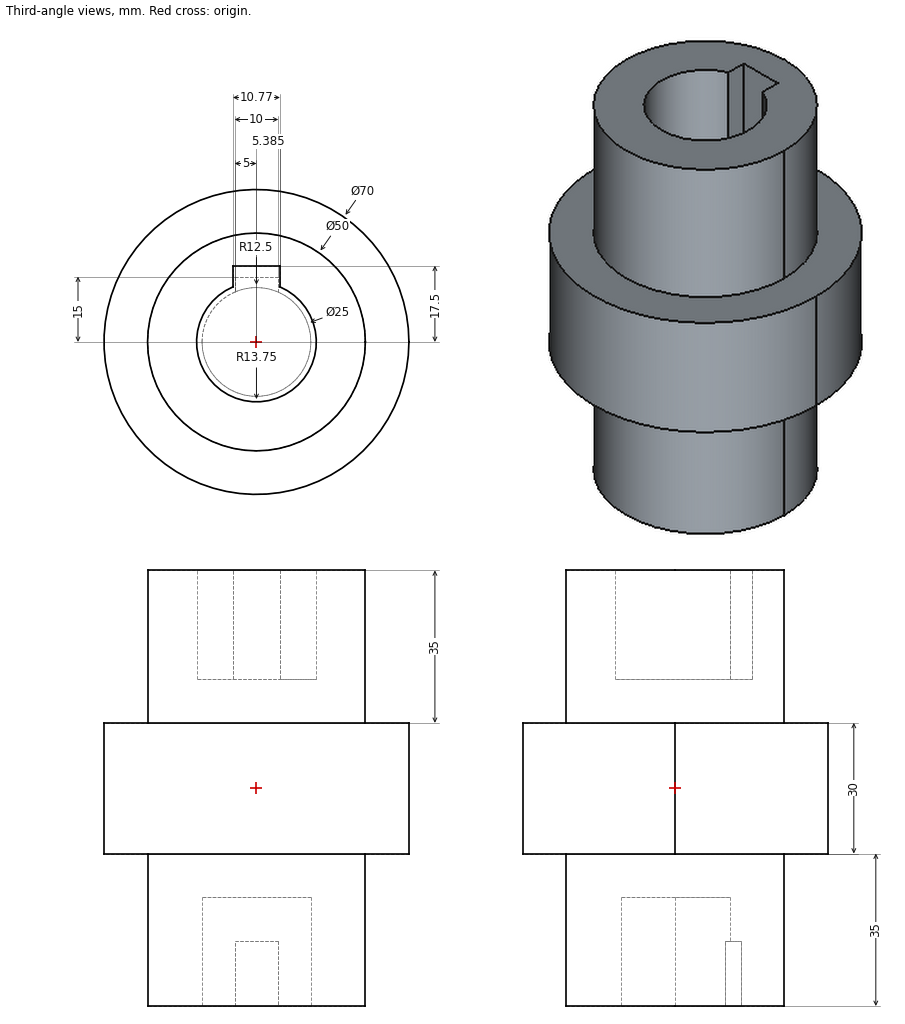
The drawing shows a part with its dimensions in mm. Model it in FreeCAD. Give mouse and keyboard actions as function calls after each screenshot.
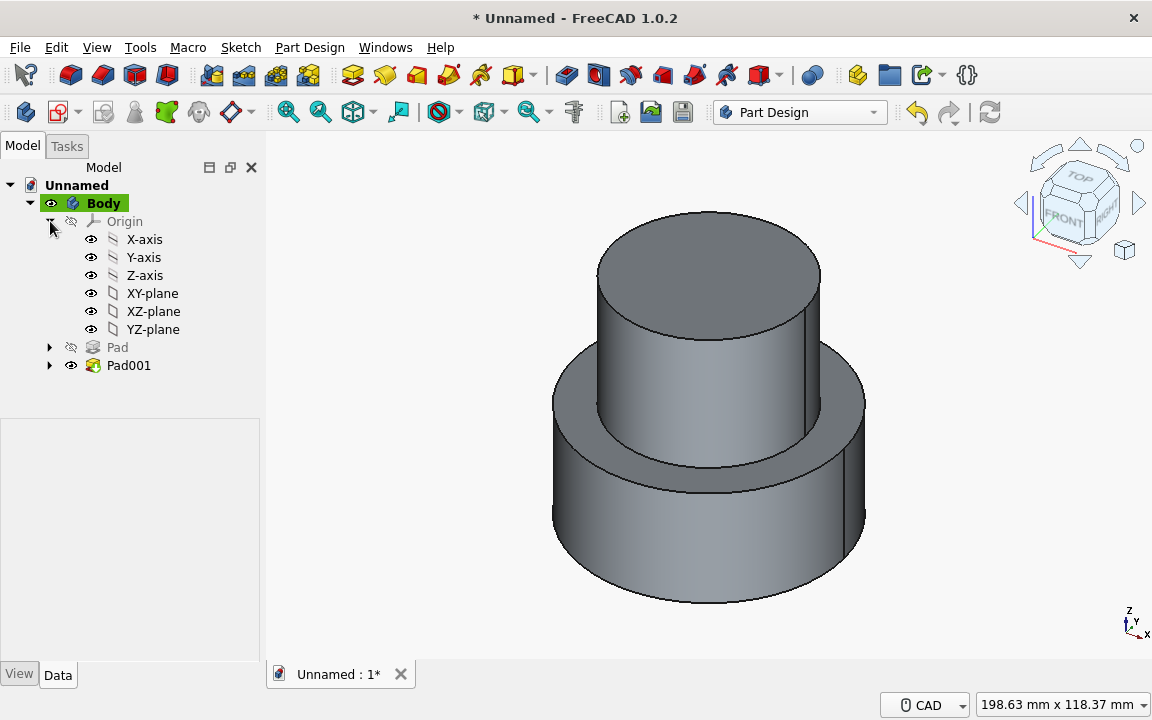
click(136, 293)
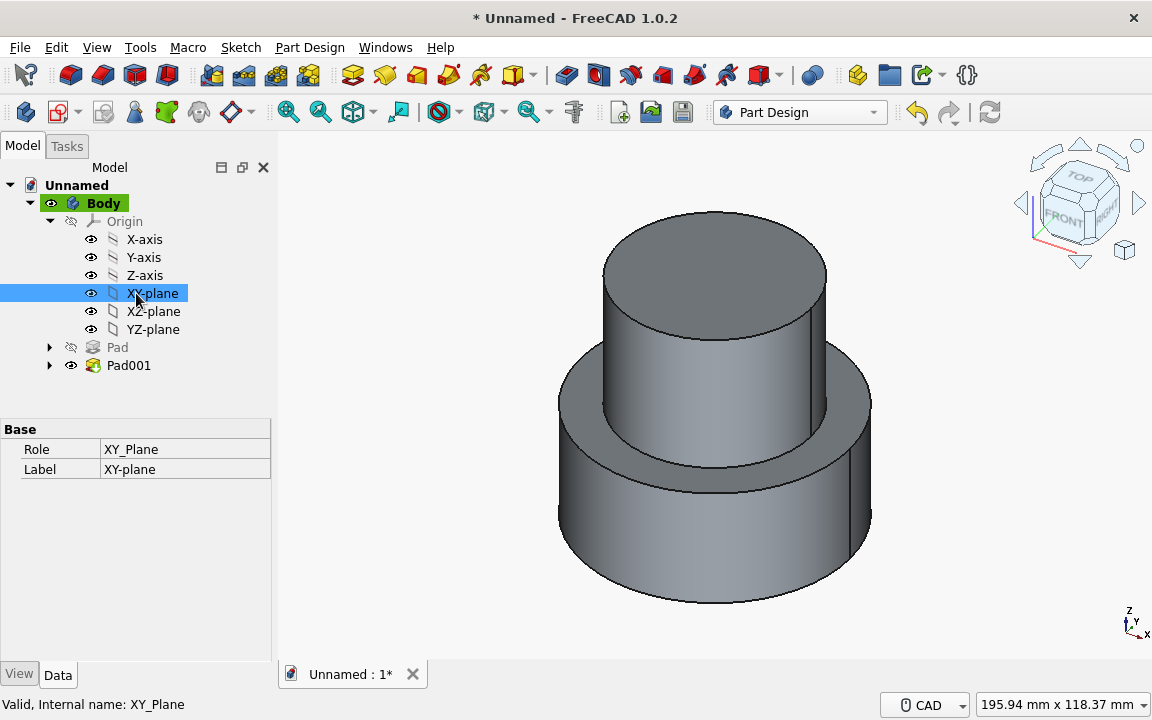
click(232, 112)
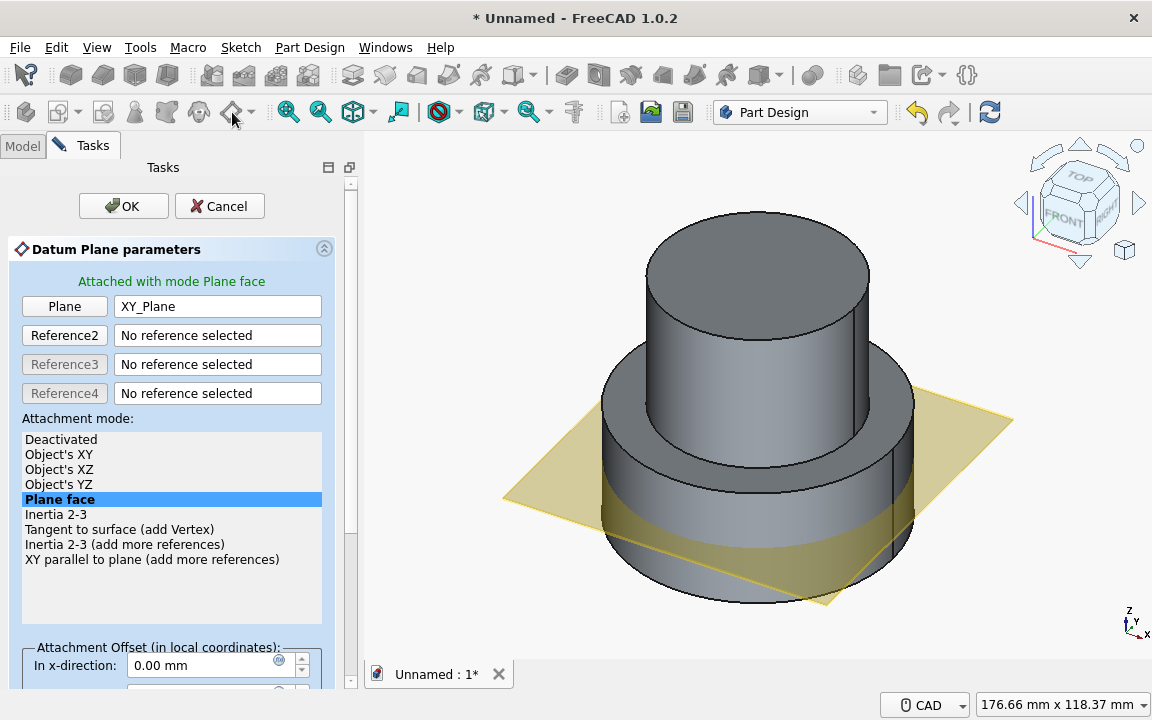
scroll(351, 432, down, 2)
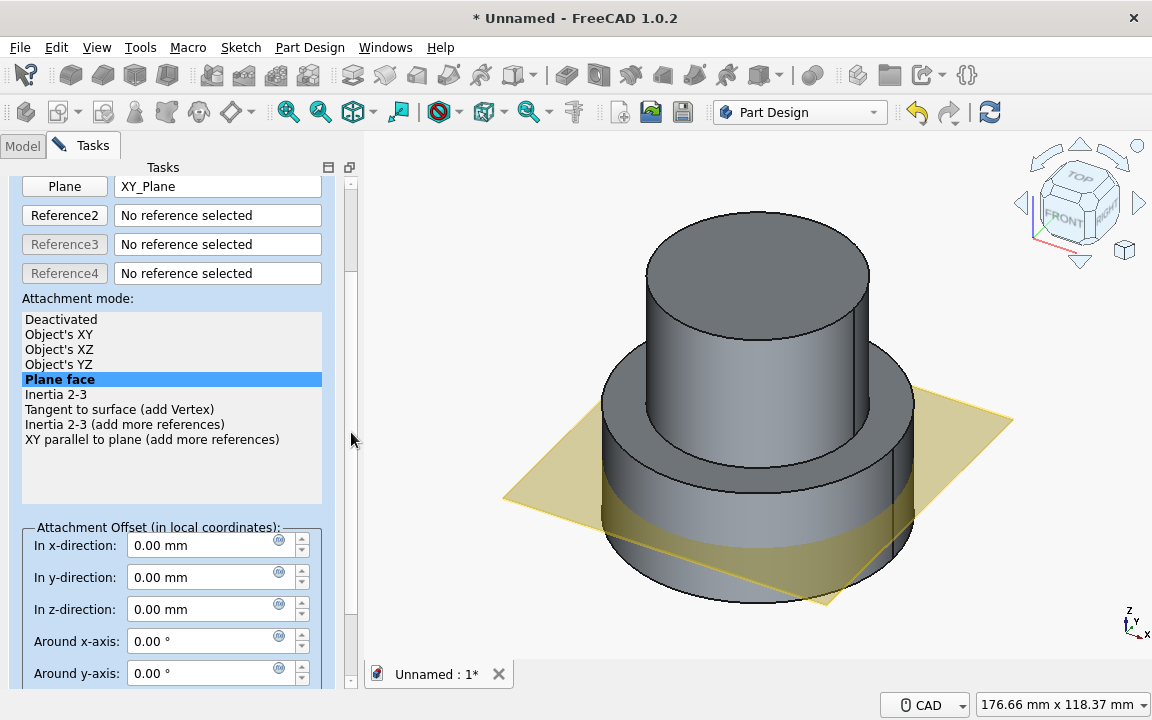
triple_click(210, 609)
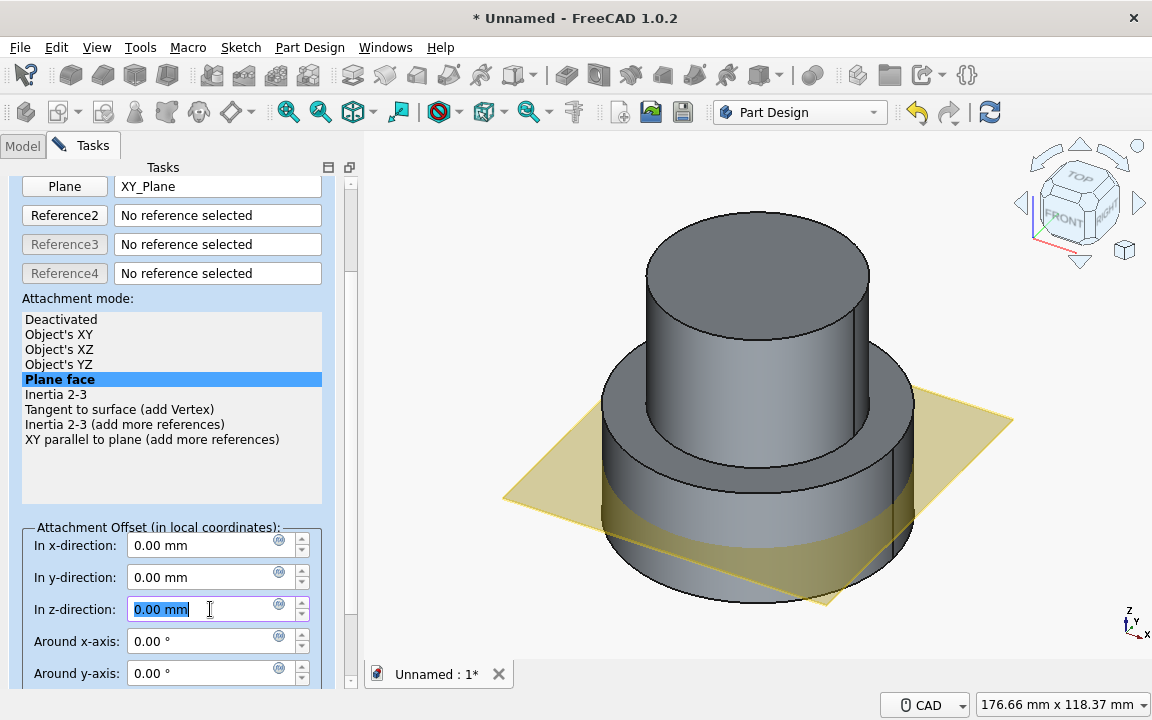
text(-50)
key(Tab)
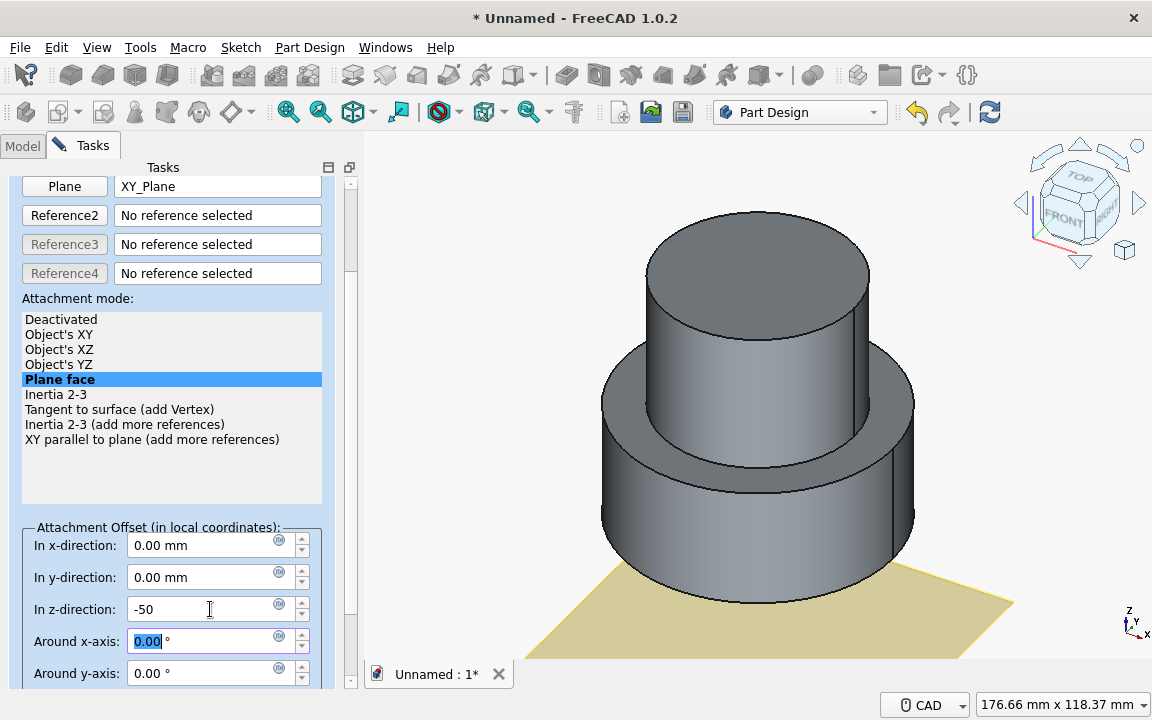
scroll(351, 432, up, 3)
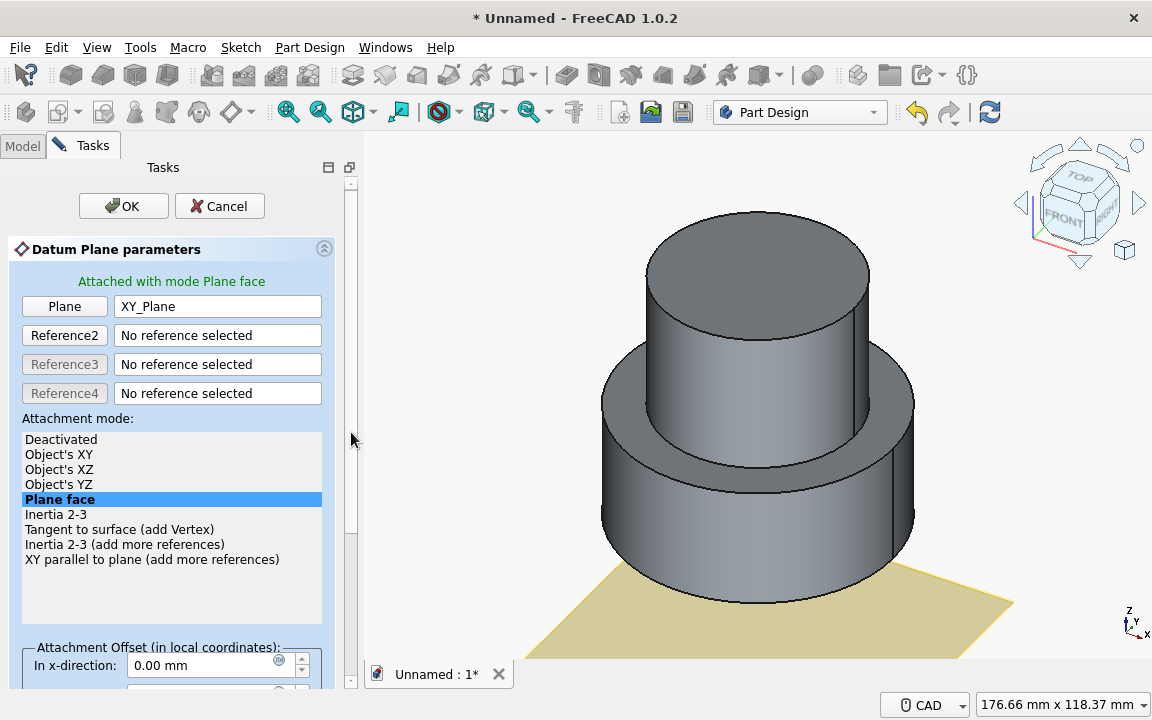
click(124, 206)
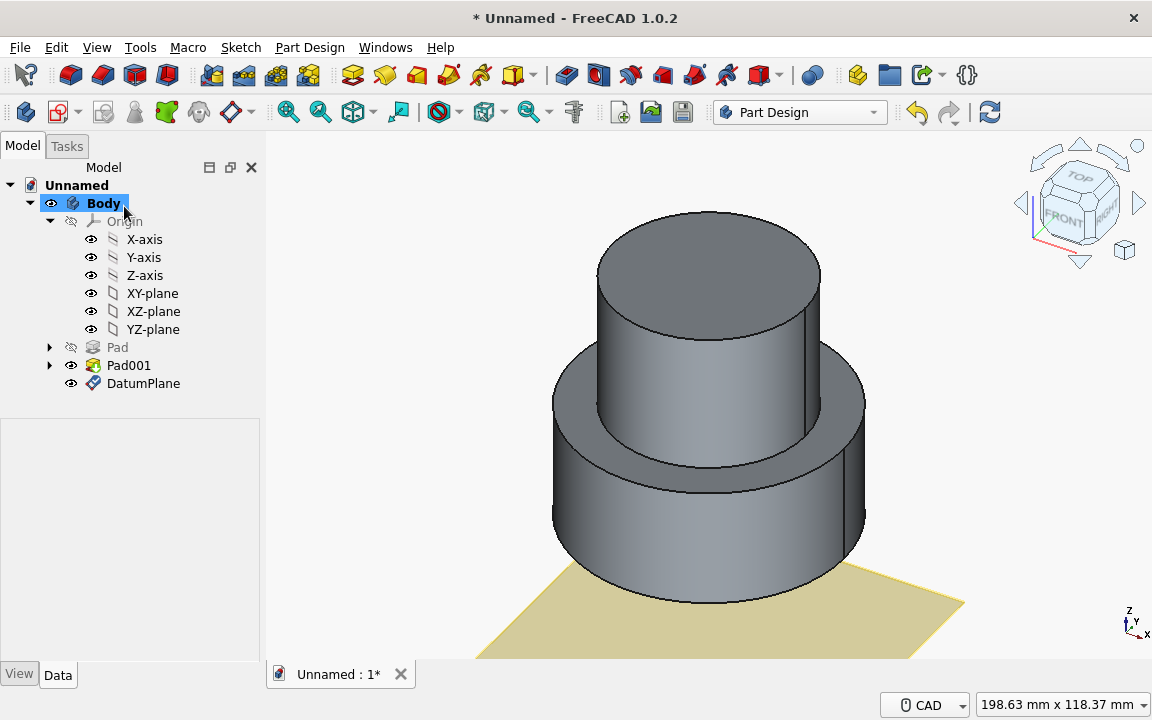
click(116, 383)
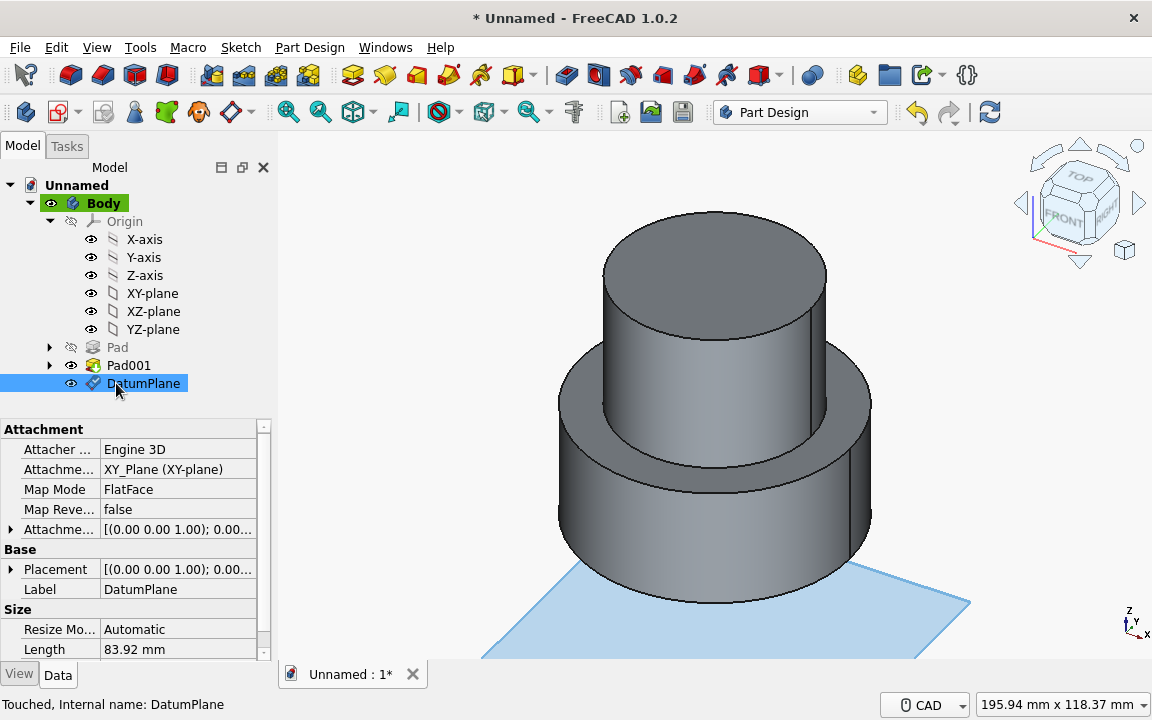
click(58, 112)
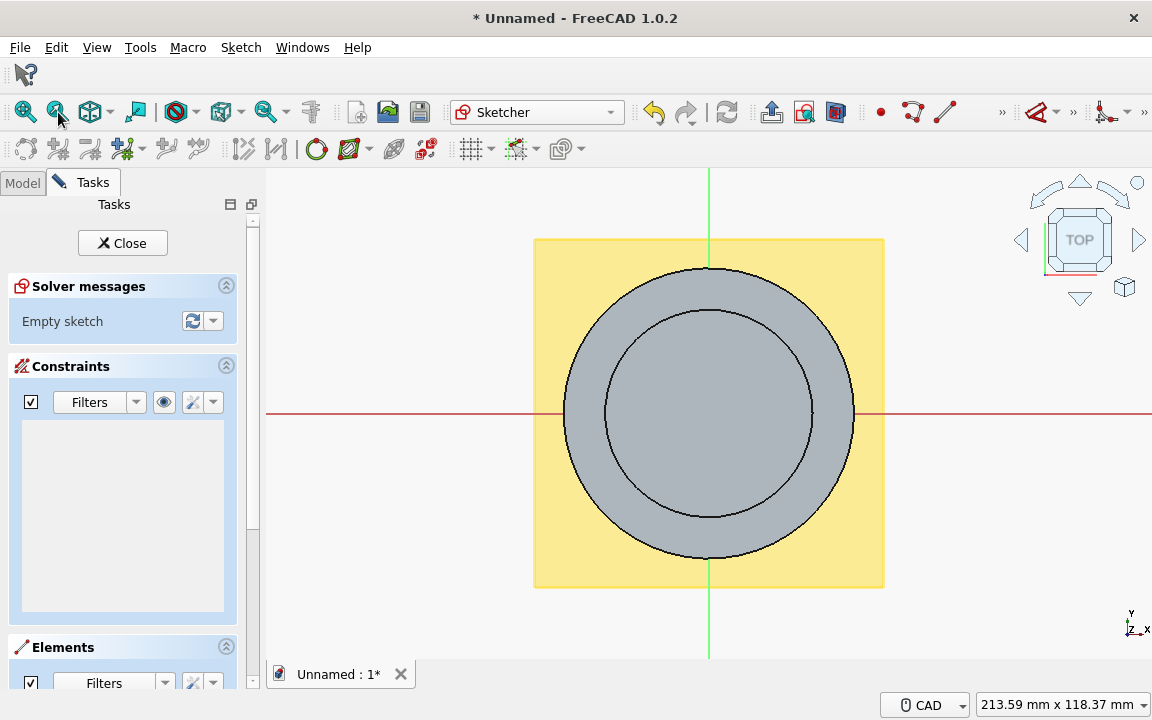
click(836, 112)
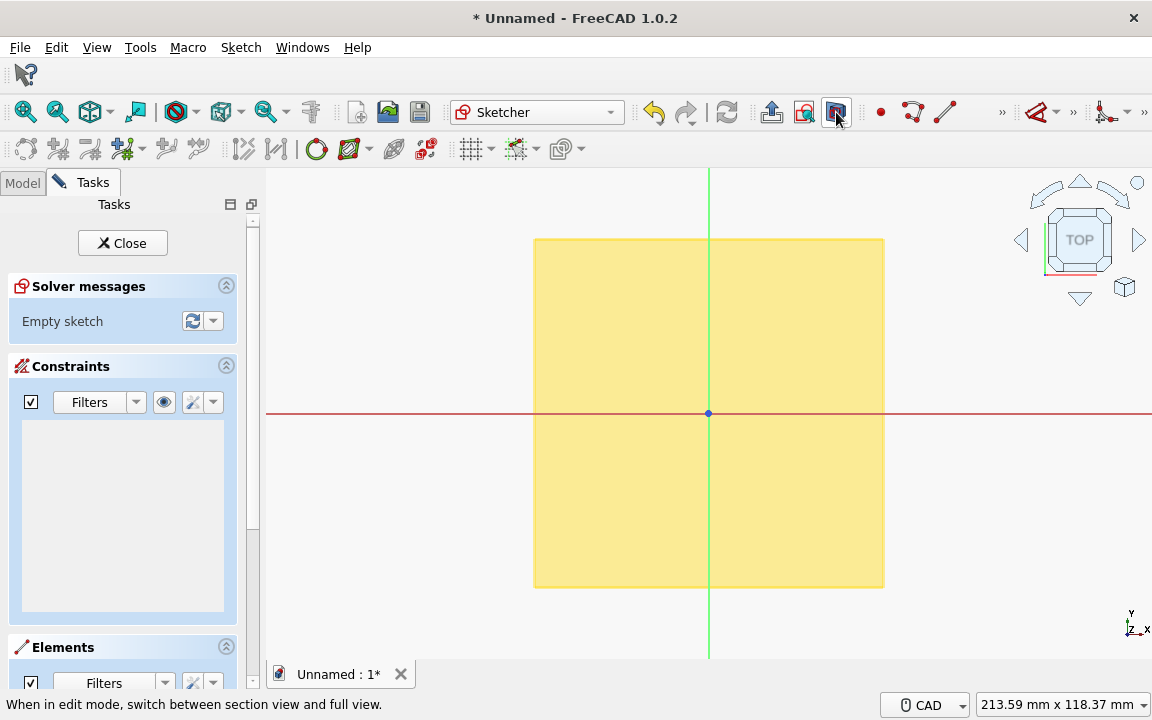
scroll(848, 413, up, 2)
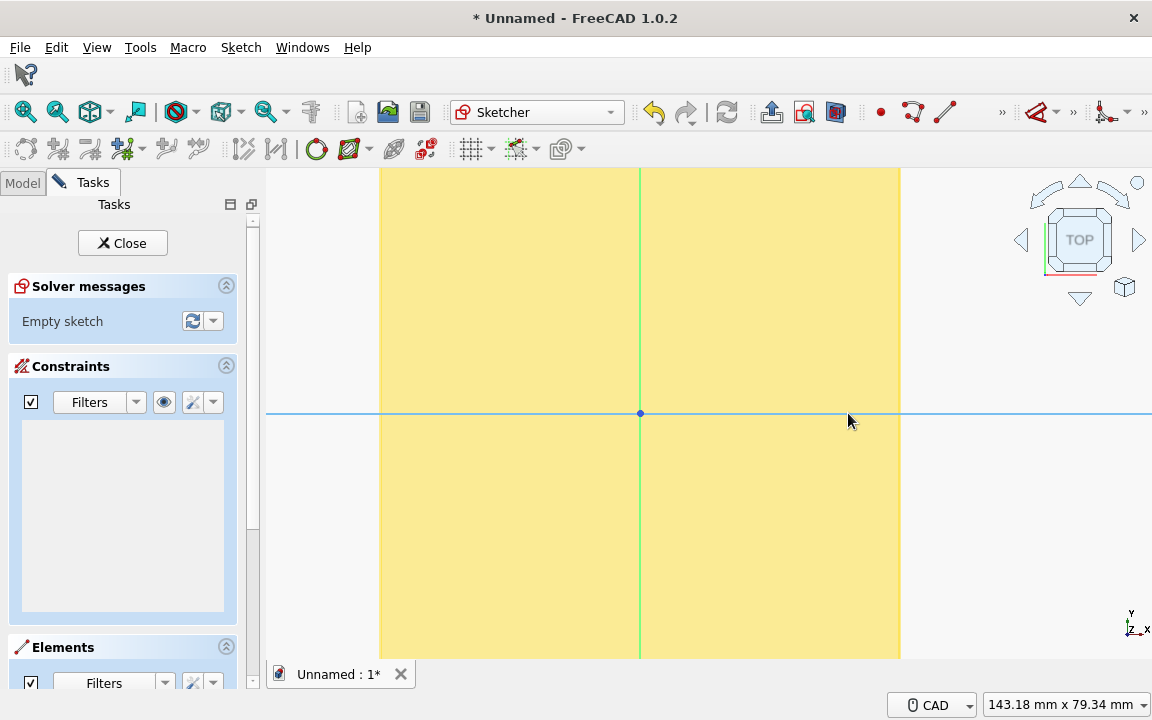
key(g)
key(c)